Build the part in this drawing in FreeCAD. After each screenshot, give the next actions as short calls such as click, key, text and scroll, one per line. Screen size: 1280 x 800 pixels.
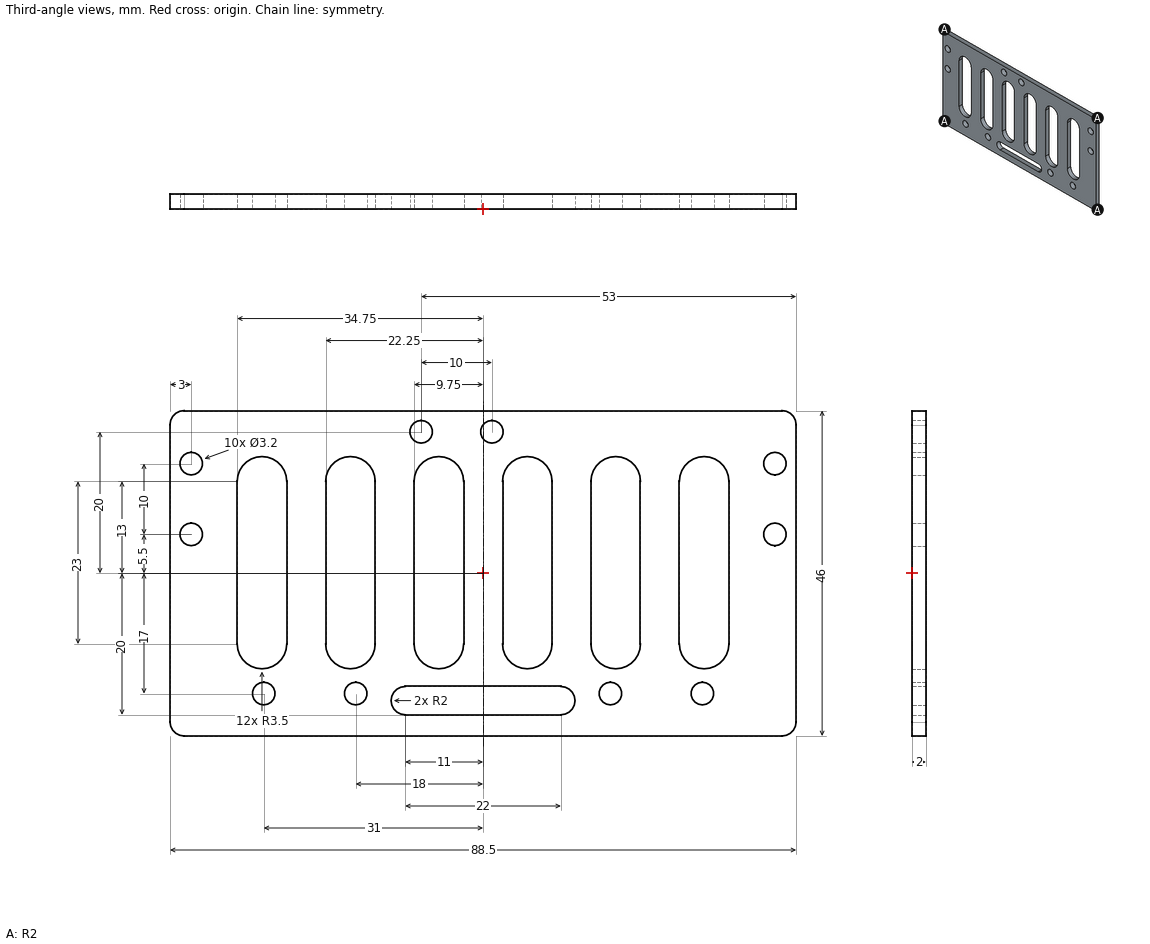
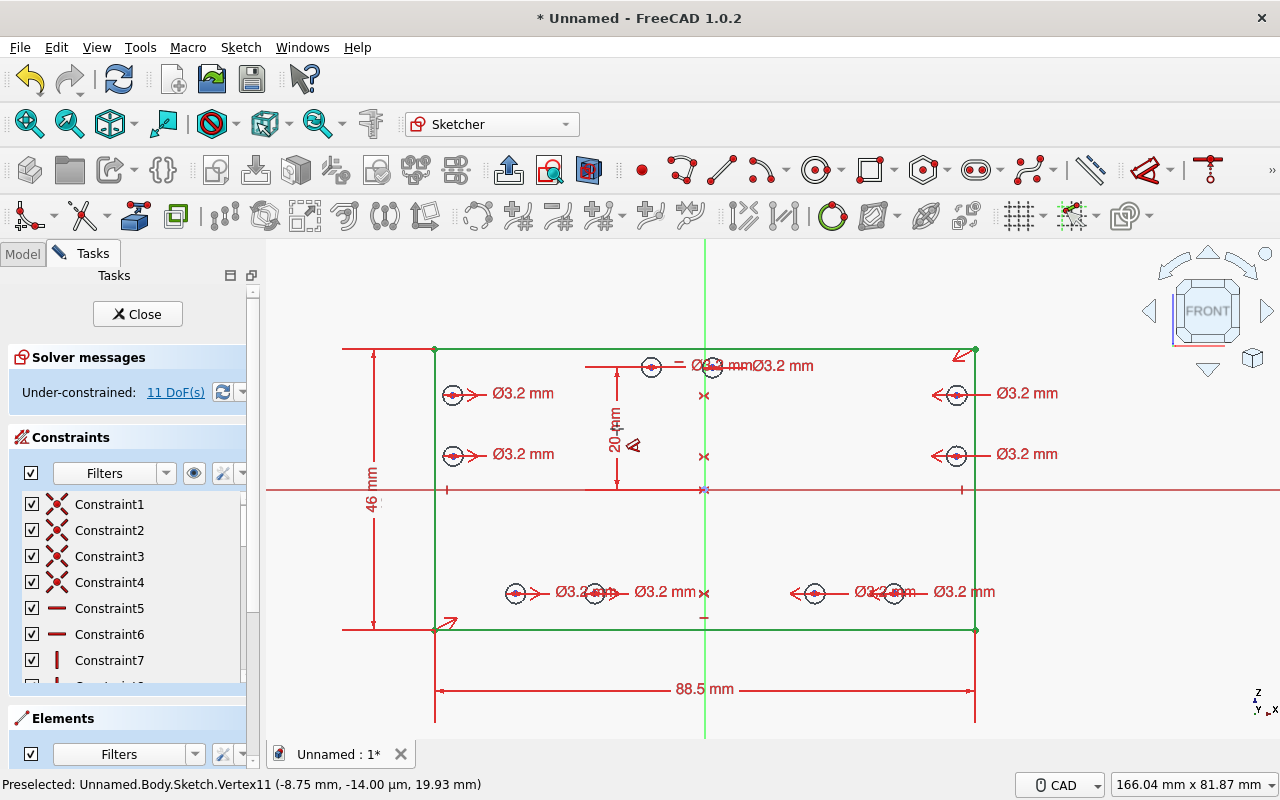
click(713, 368)
click(747, 429)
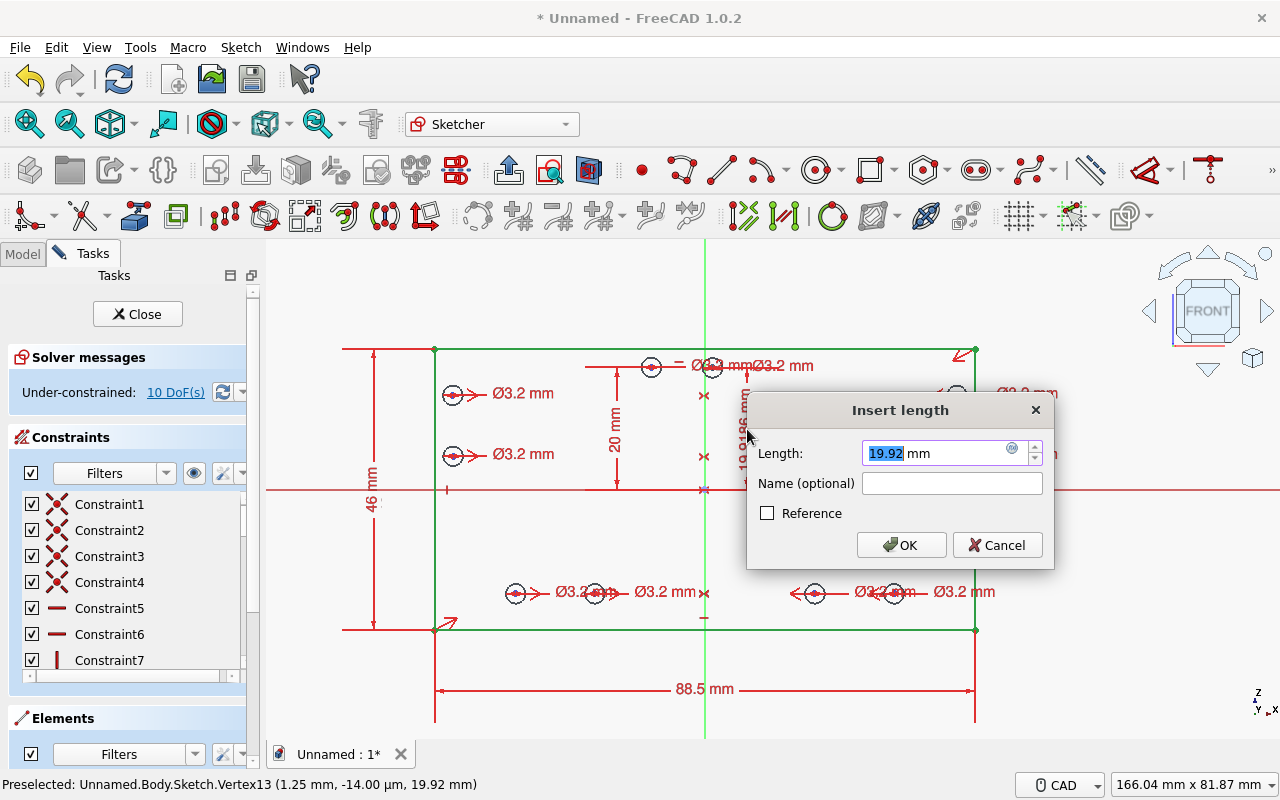
text(20)
key(Return)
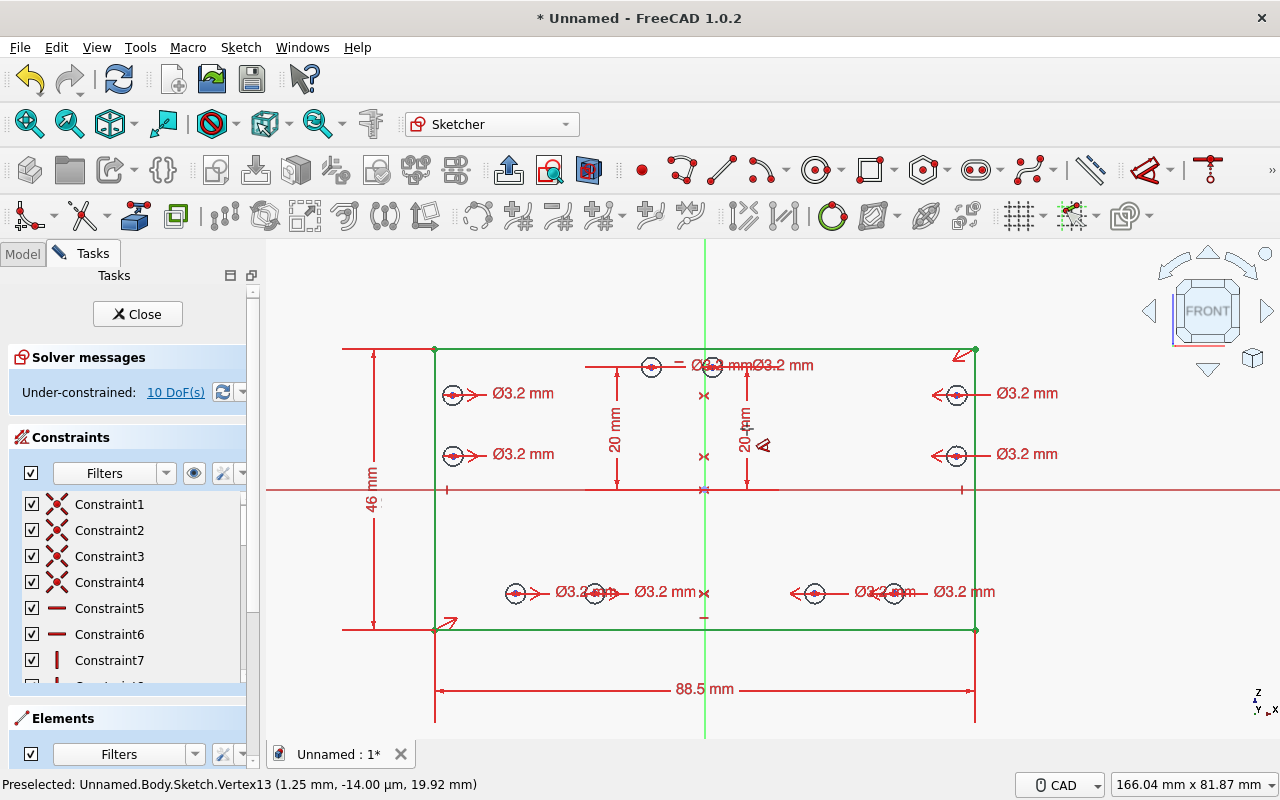
click(516, 594)
click(610, 456)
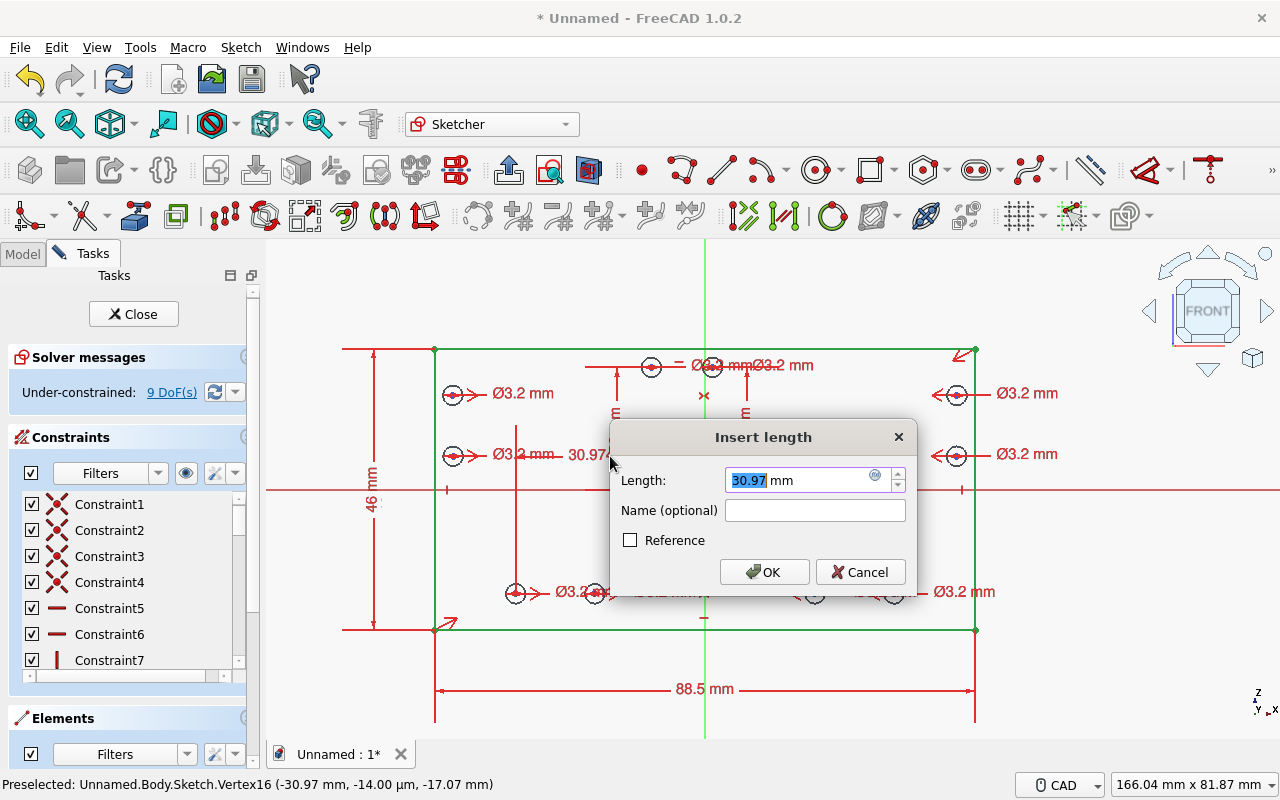
text(31)
key(Return)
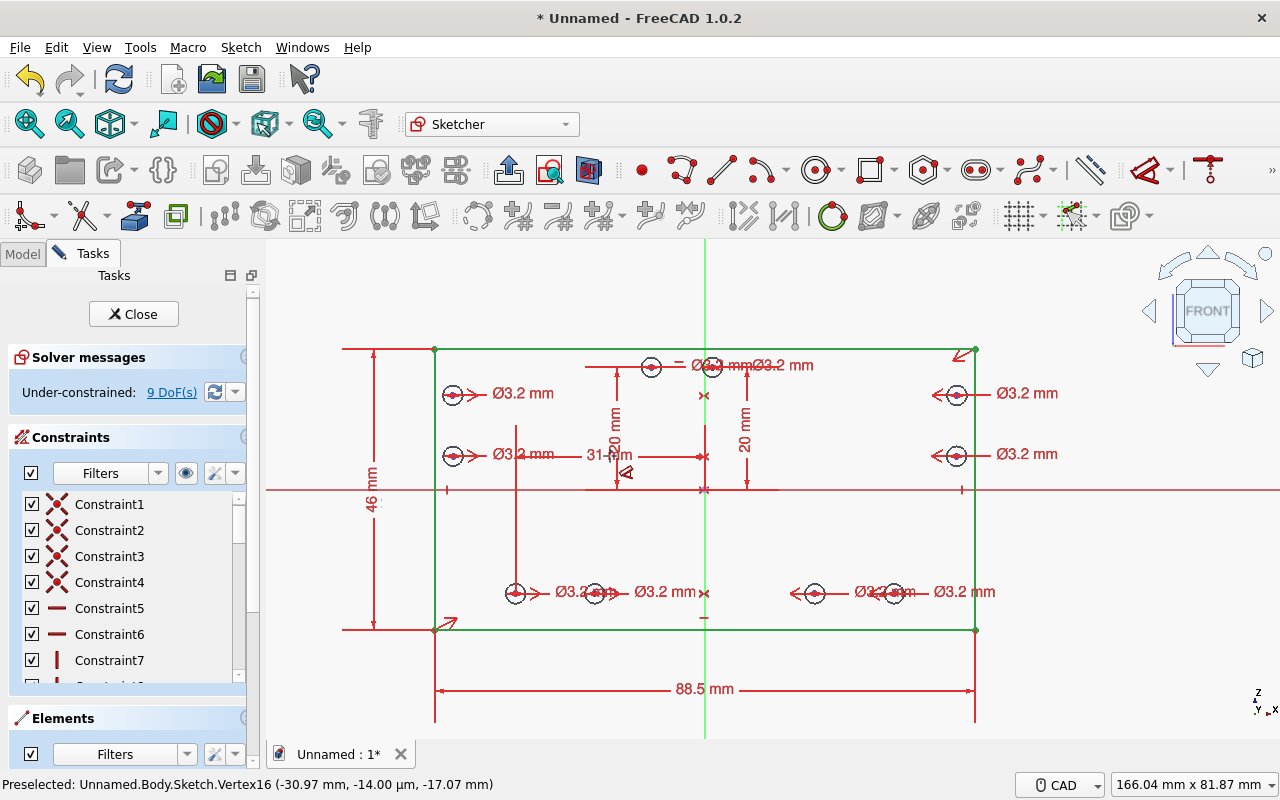
click(516, 594)
click(482, 542)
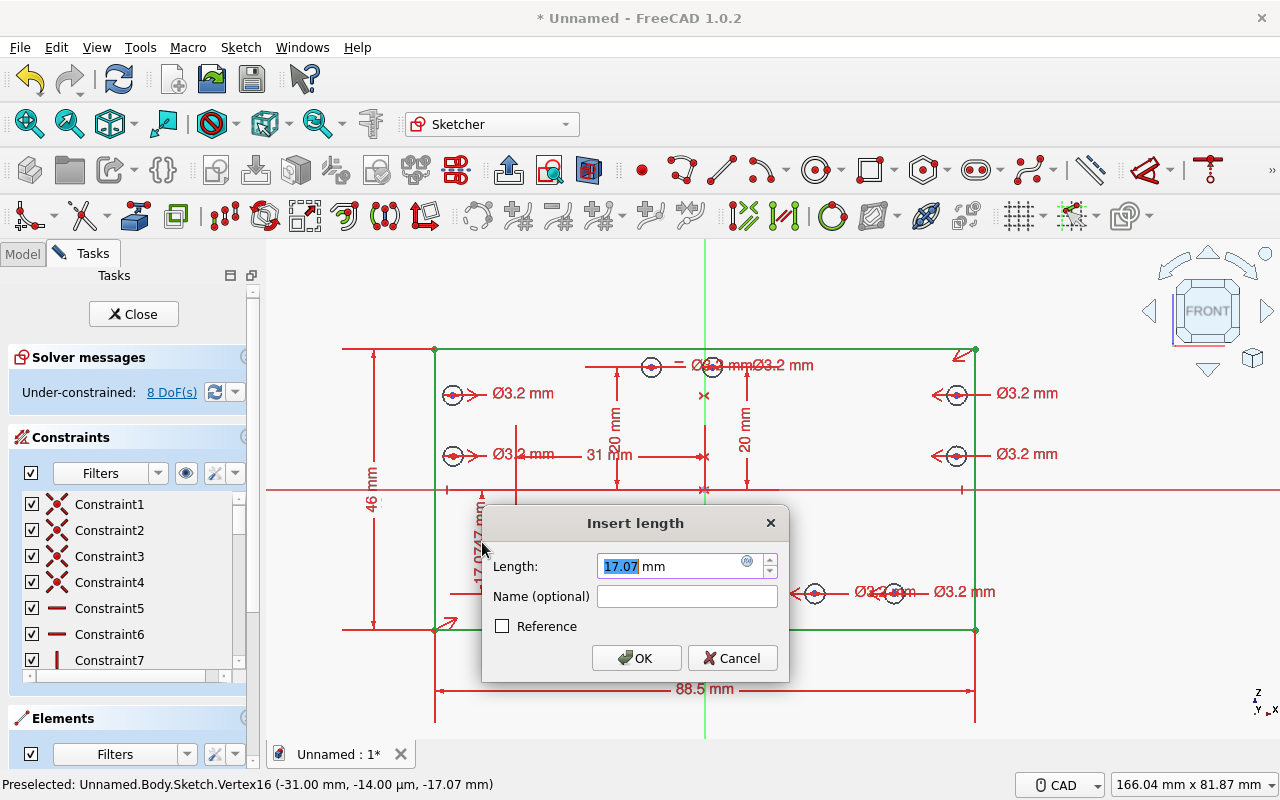
text(17)
key(Return)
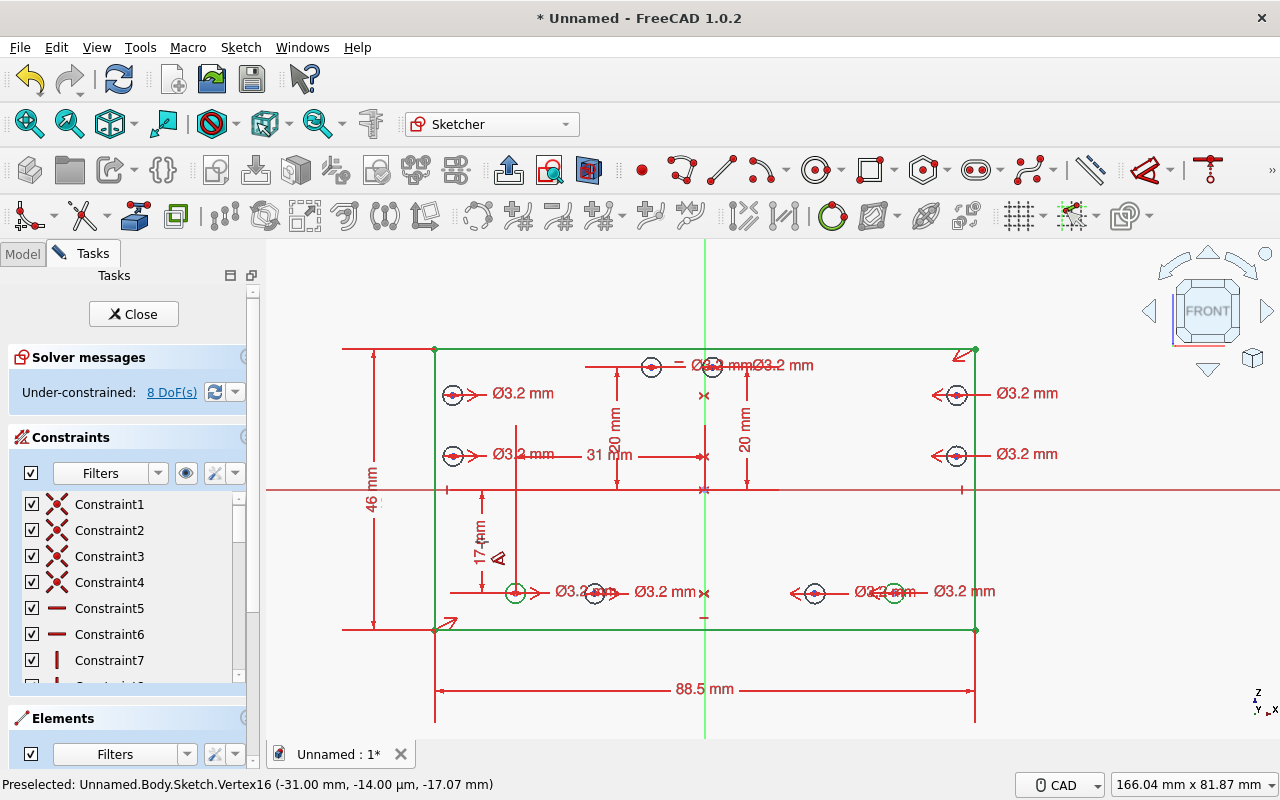
click(595, 594)
click(688, 456)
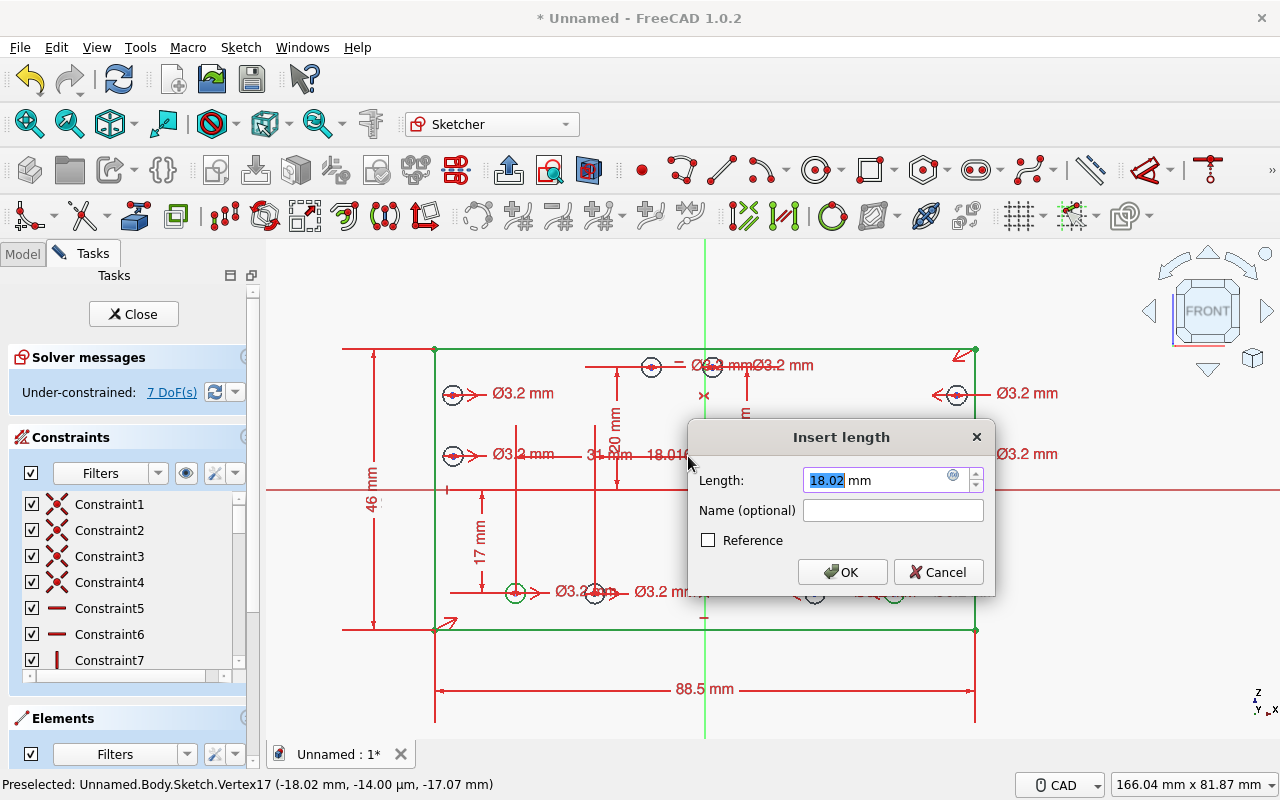
text(18)
key(Return)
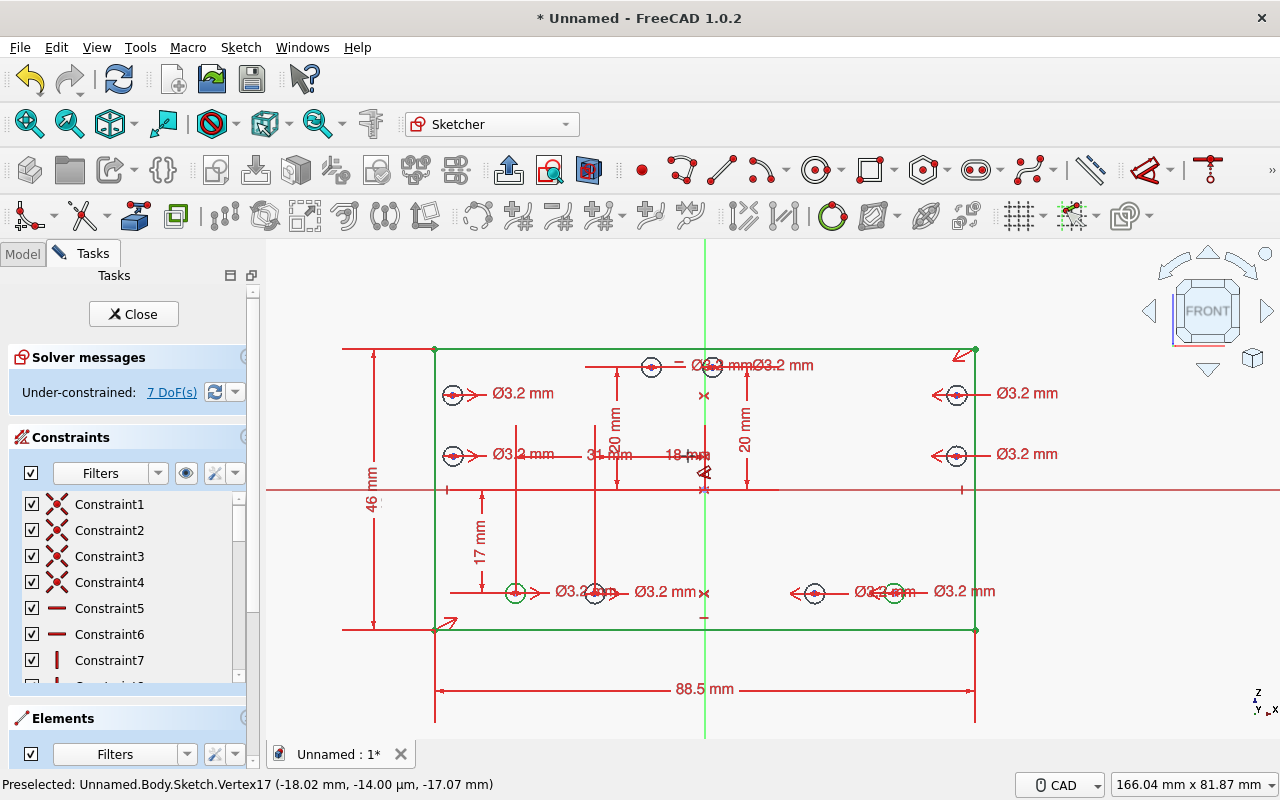
click(595, 594)
click(561, 542)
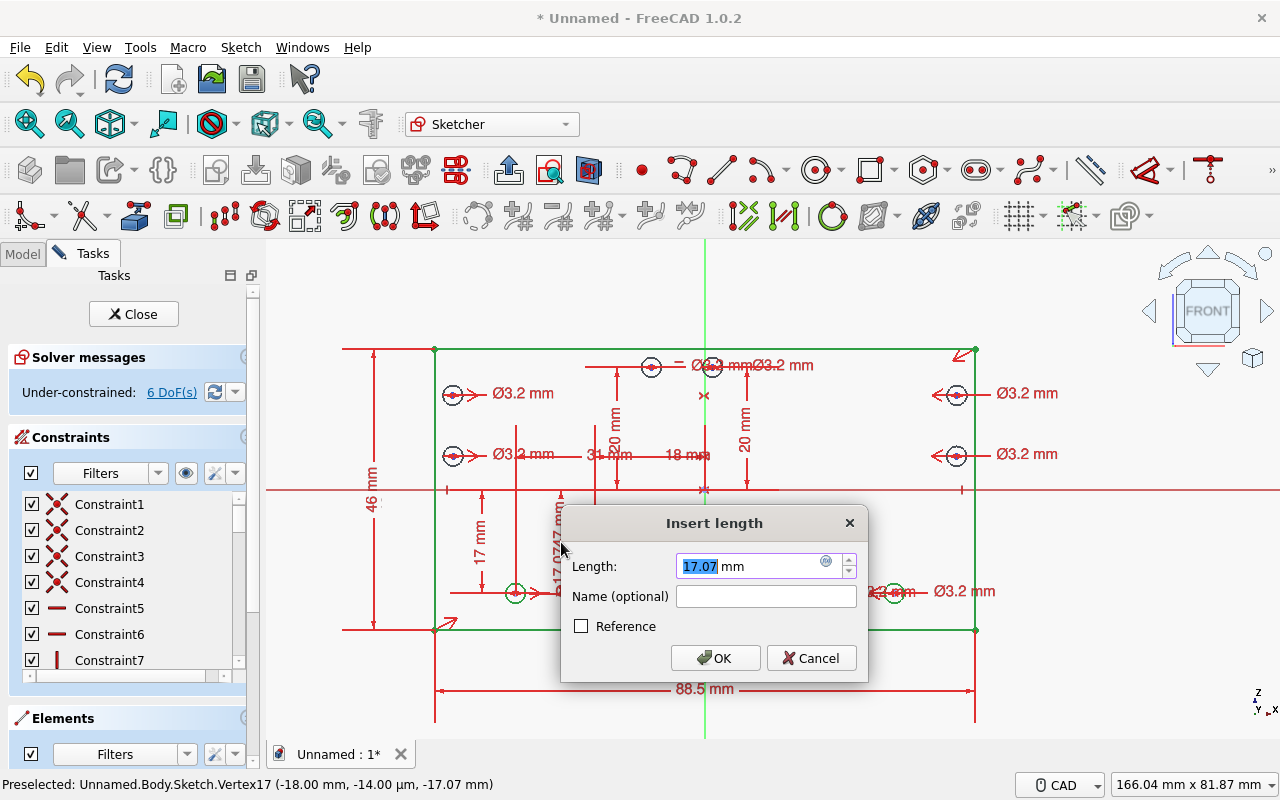
text(17)
key(Return)